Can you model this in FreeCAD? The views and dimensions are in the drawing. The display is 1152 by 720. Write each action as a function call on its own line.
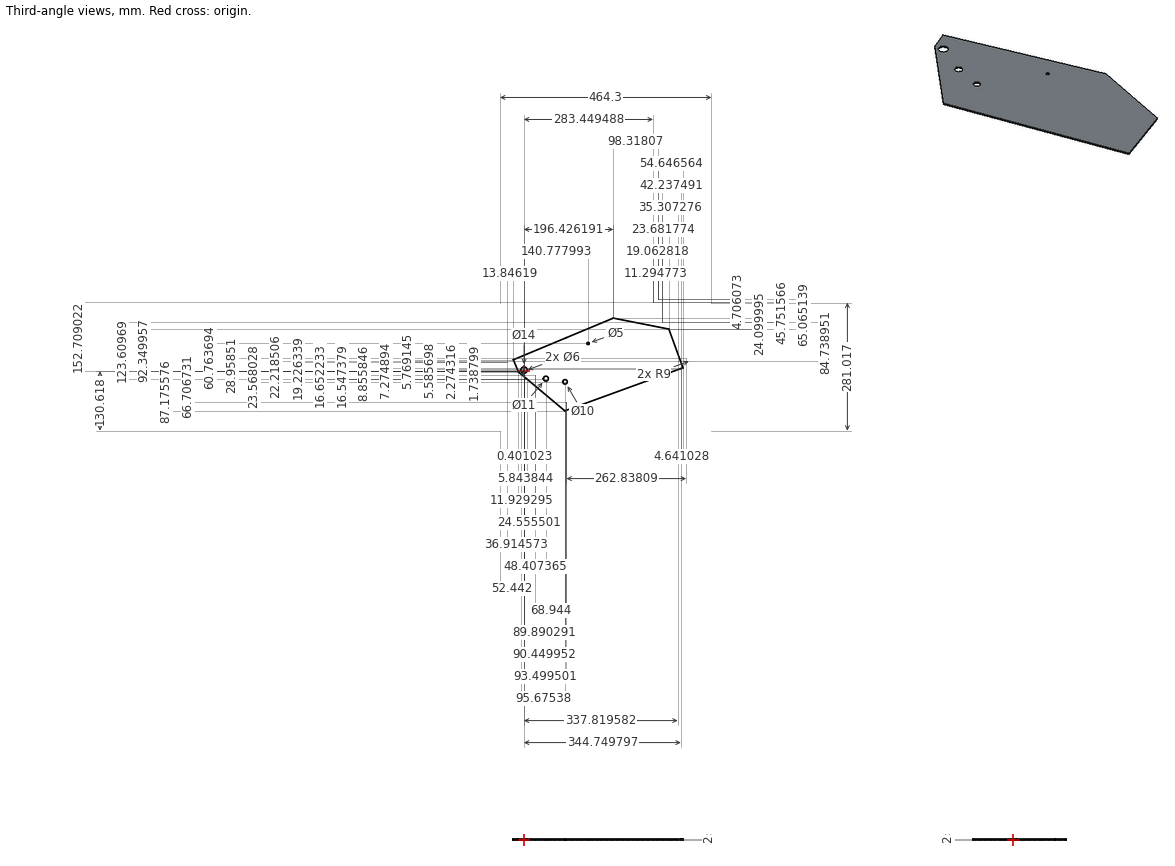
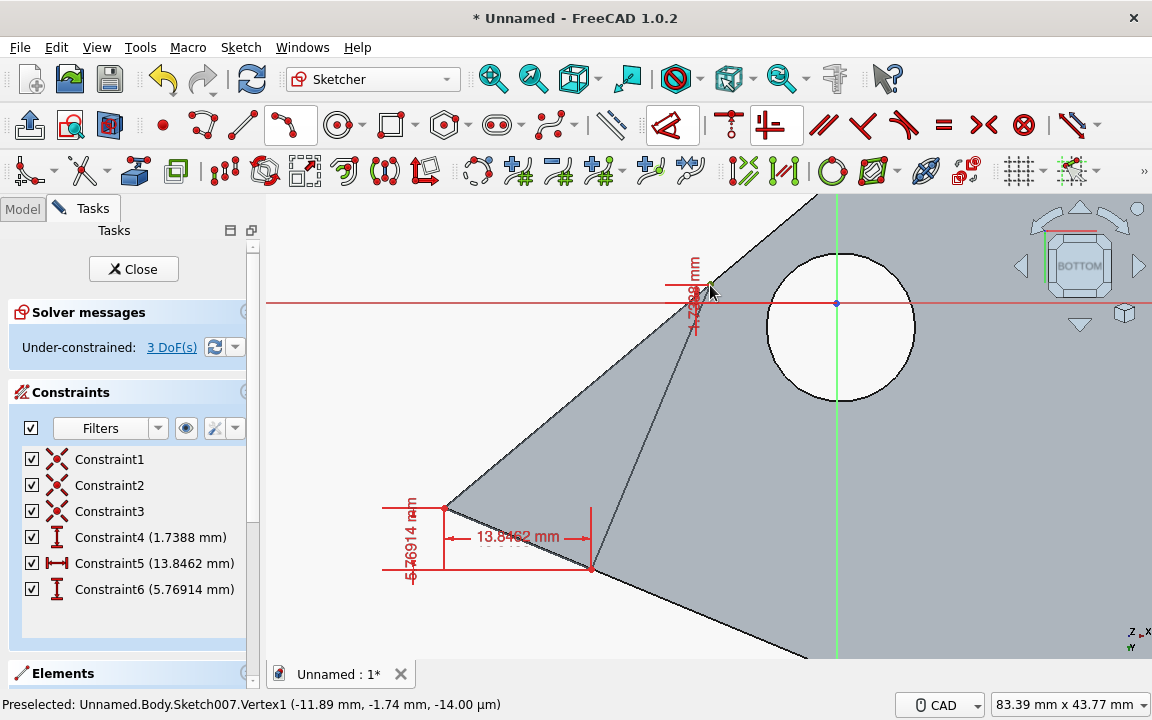
click(694, 126)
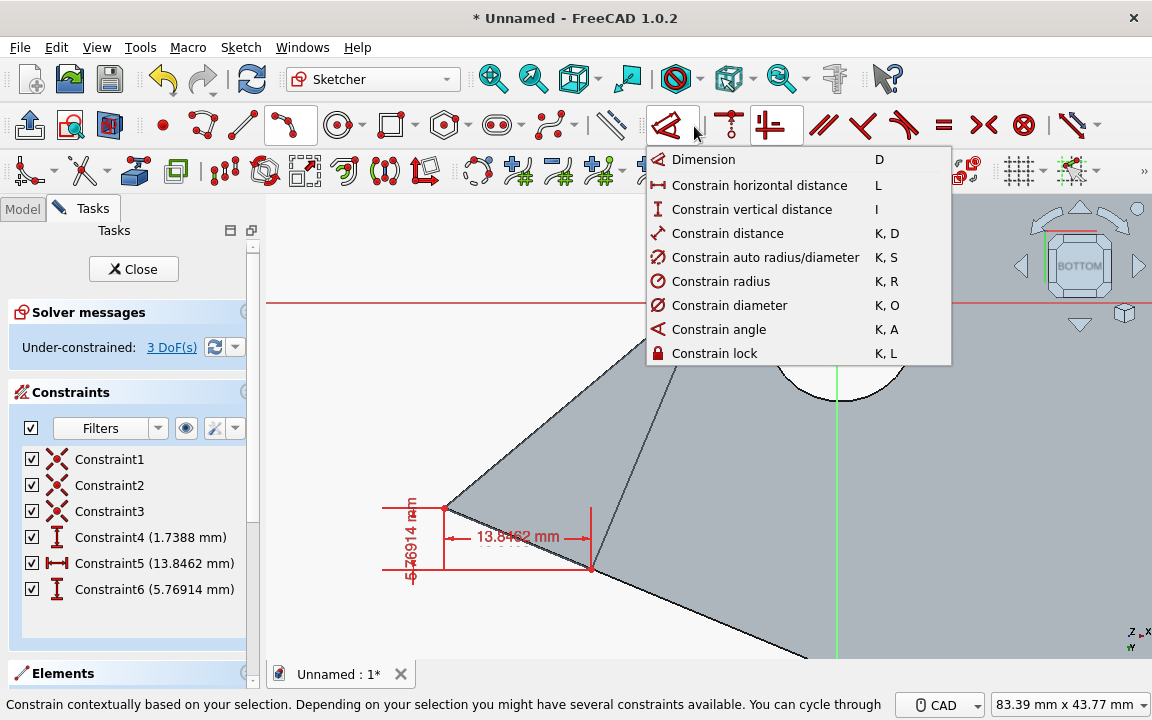
click(799, 185)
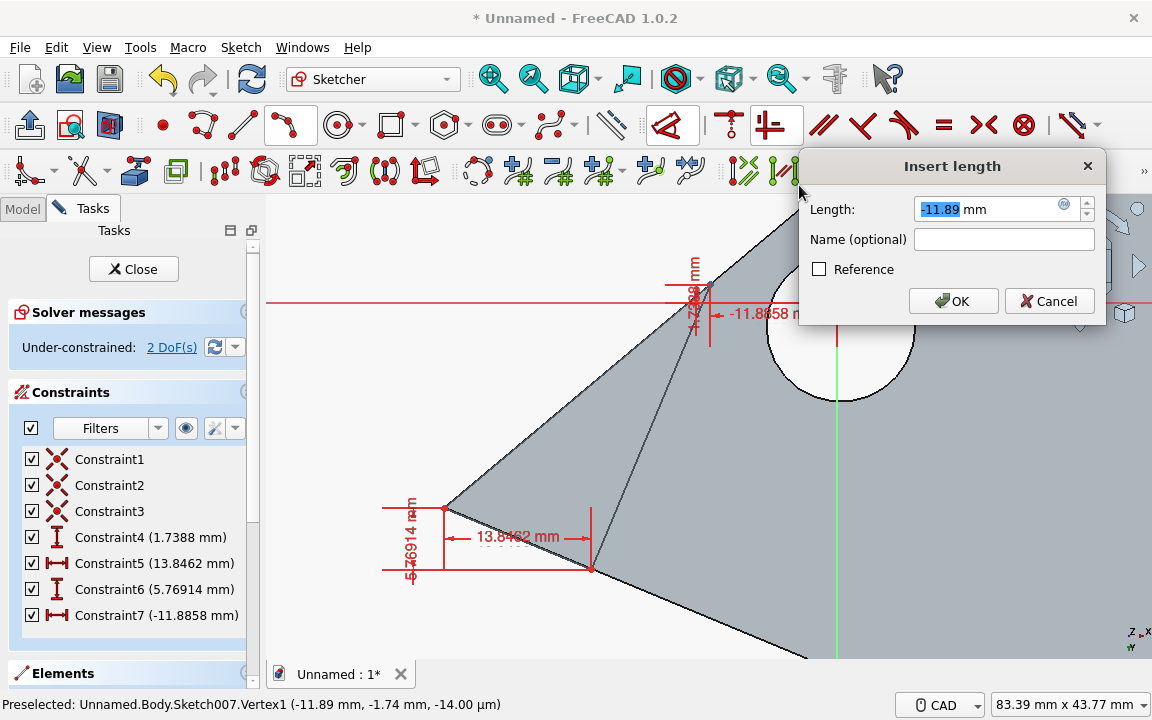
text(-11.929295)
key(Return)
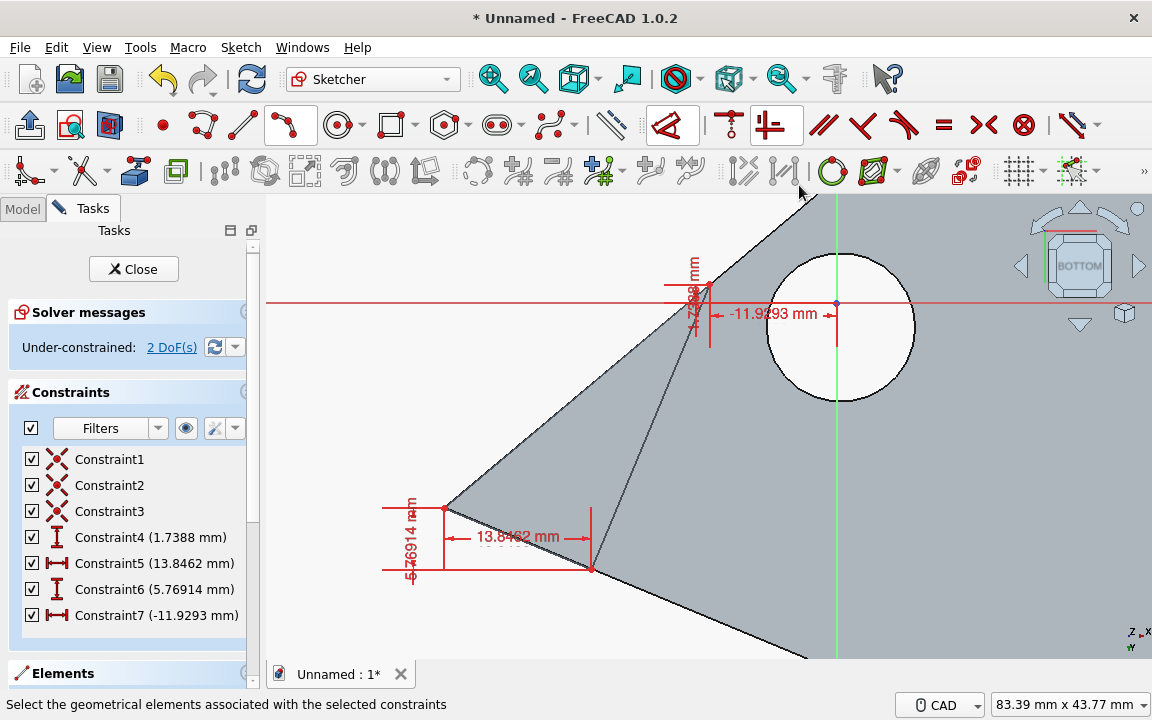
click(444, 508)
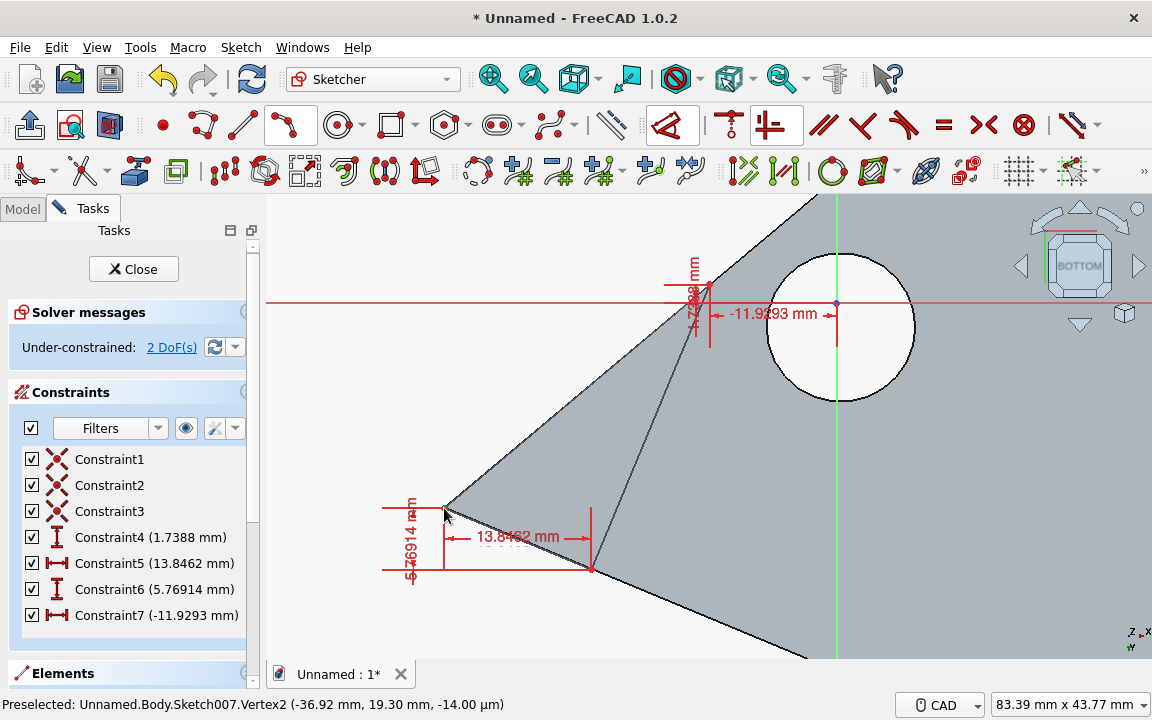
key(l)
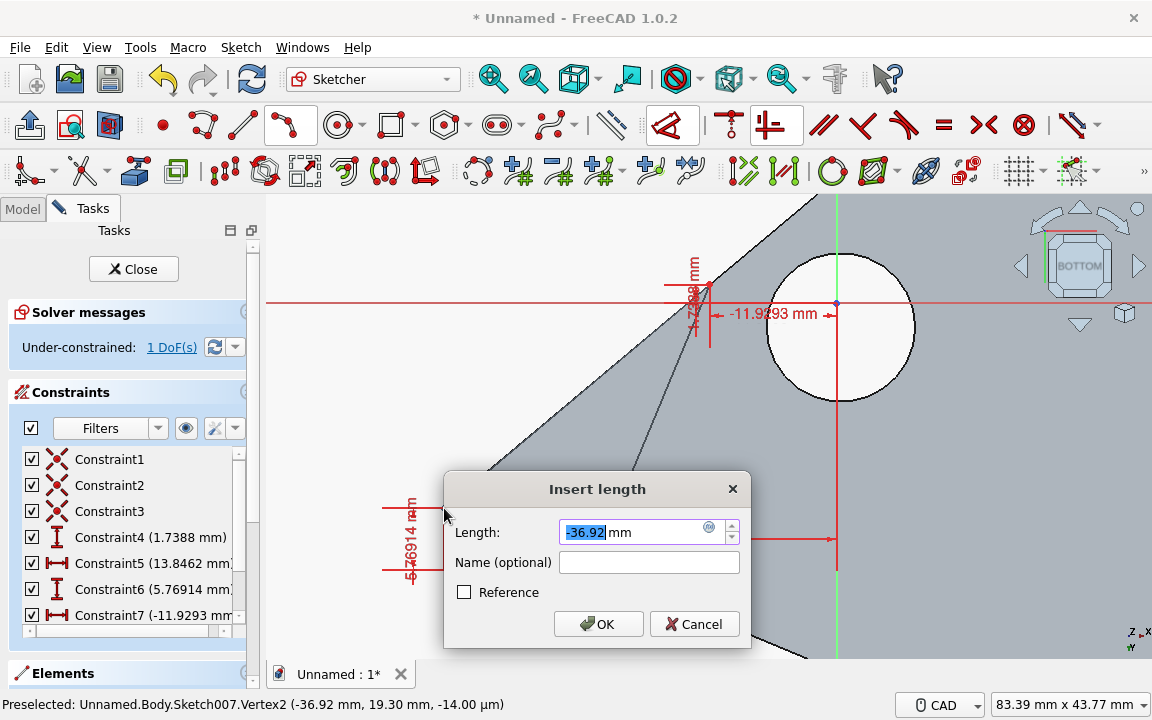
text(-36.914573)
key(Return)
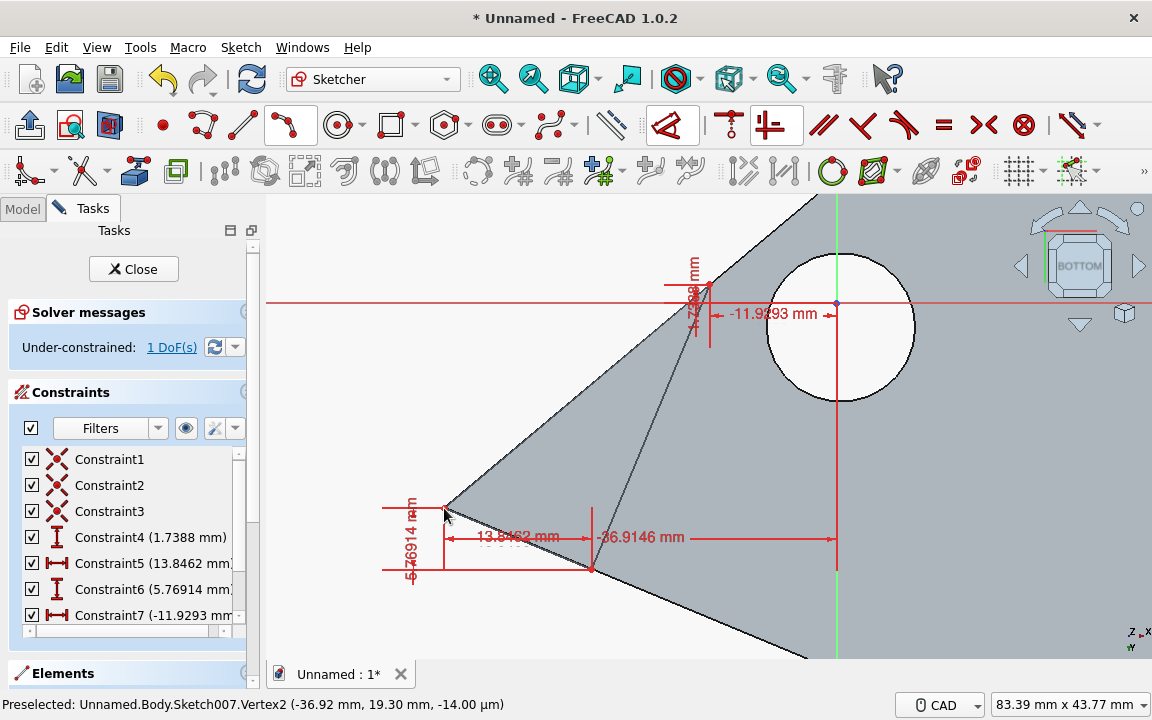
click(444, 508)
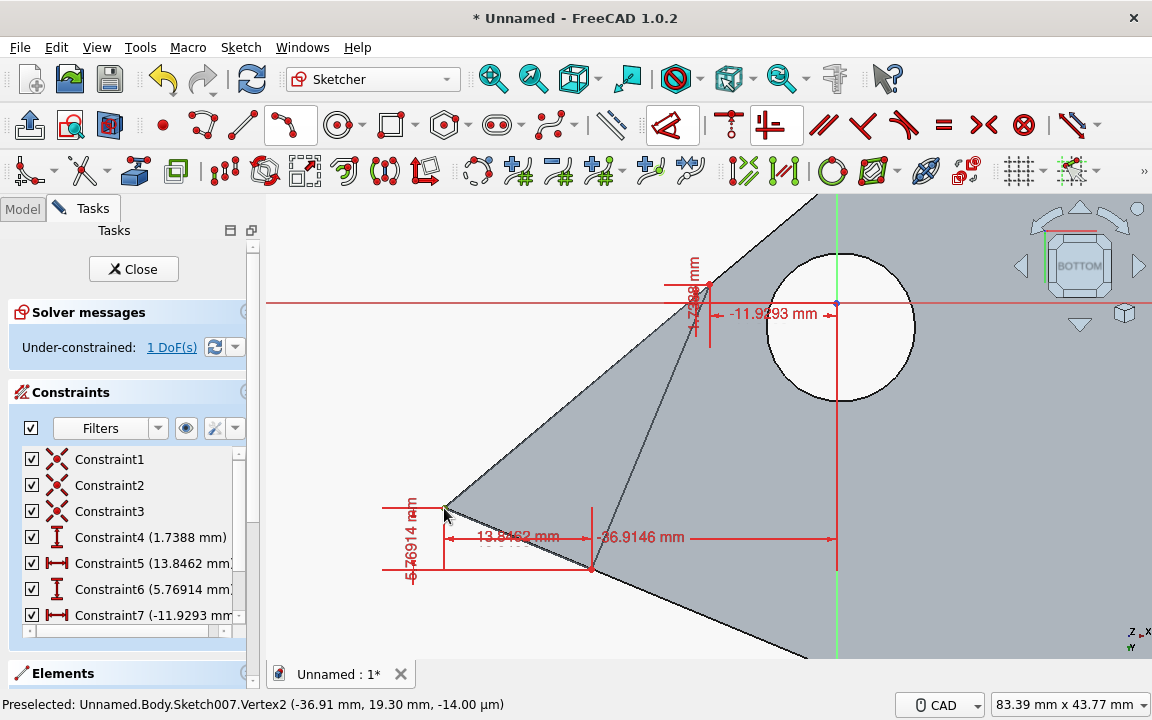
key(i)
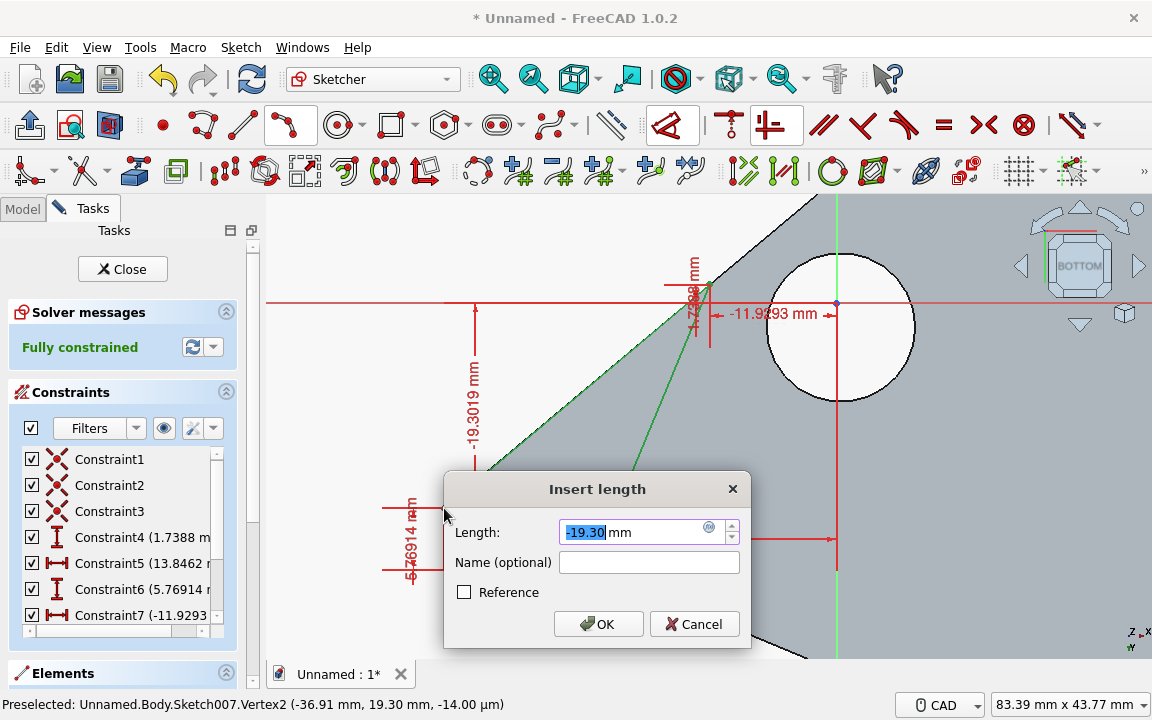
text(-19.226339)
key(Return)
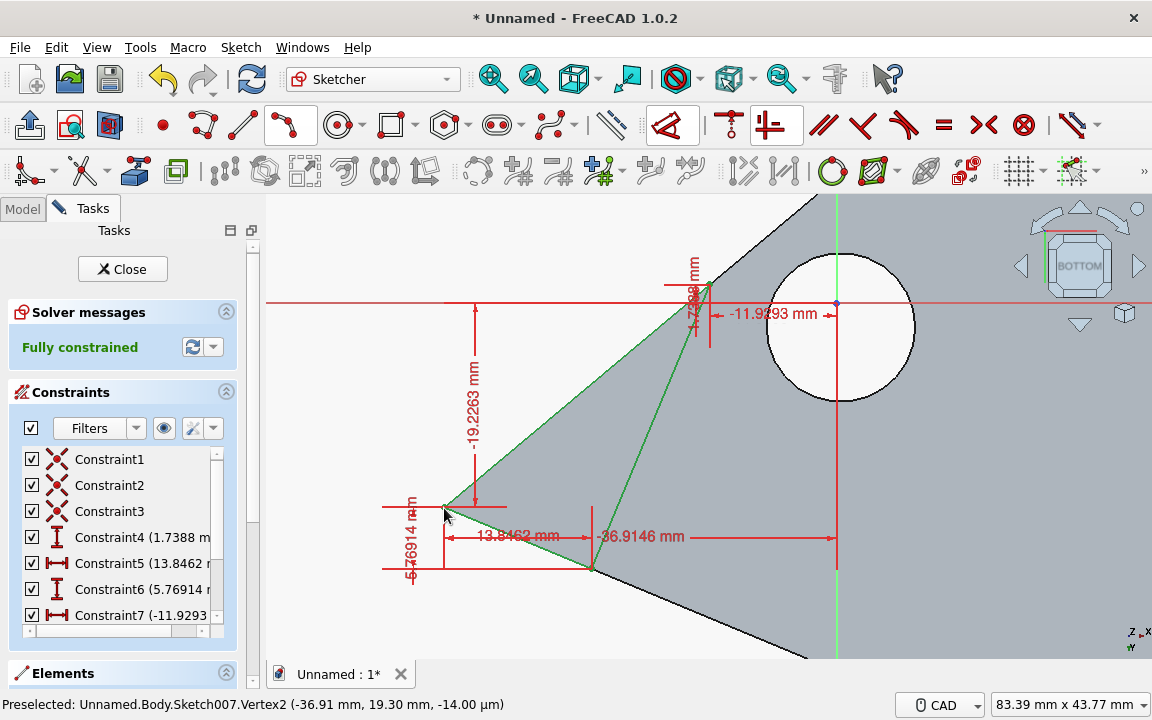
click(123, 269)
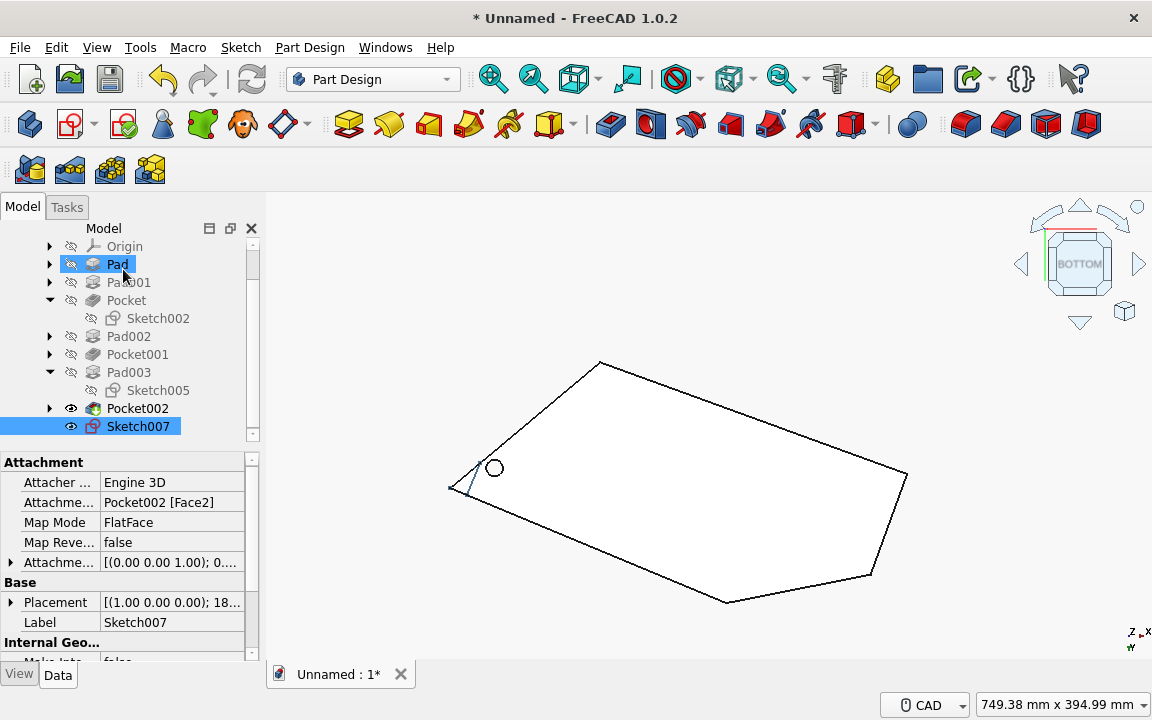
click(612, 124)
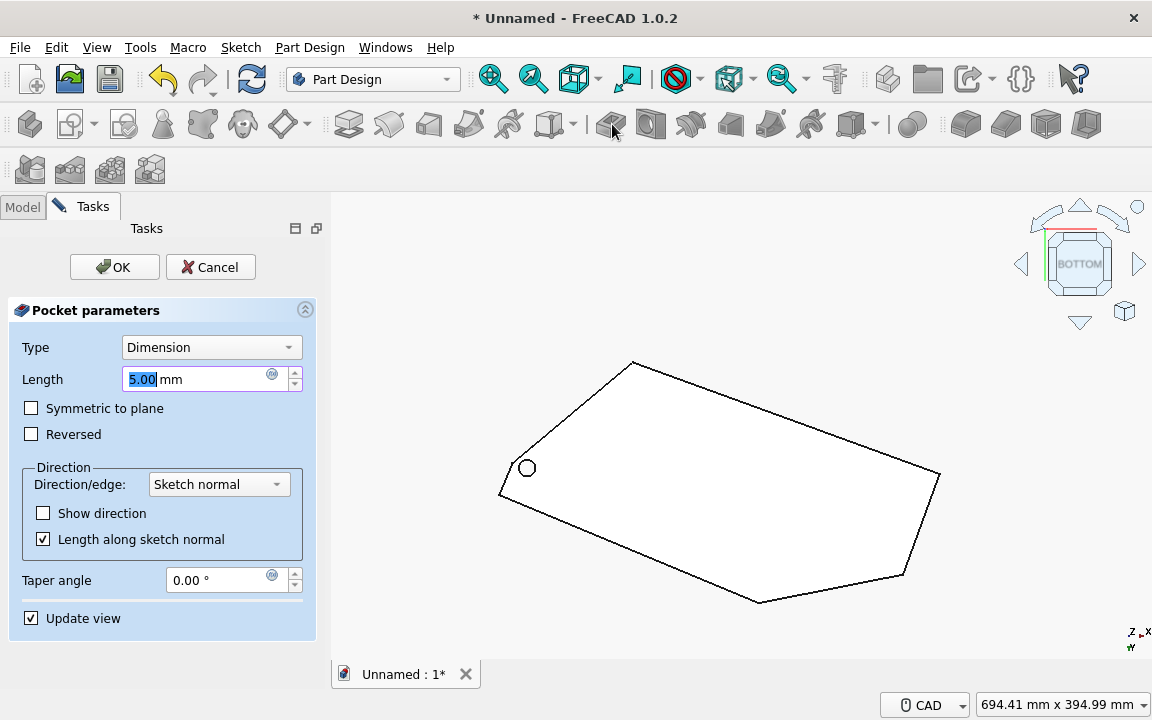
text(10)
key(Tab)